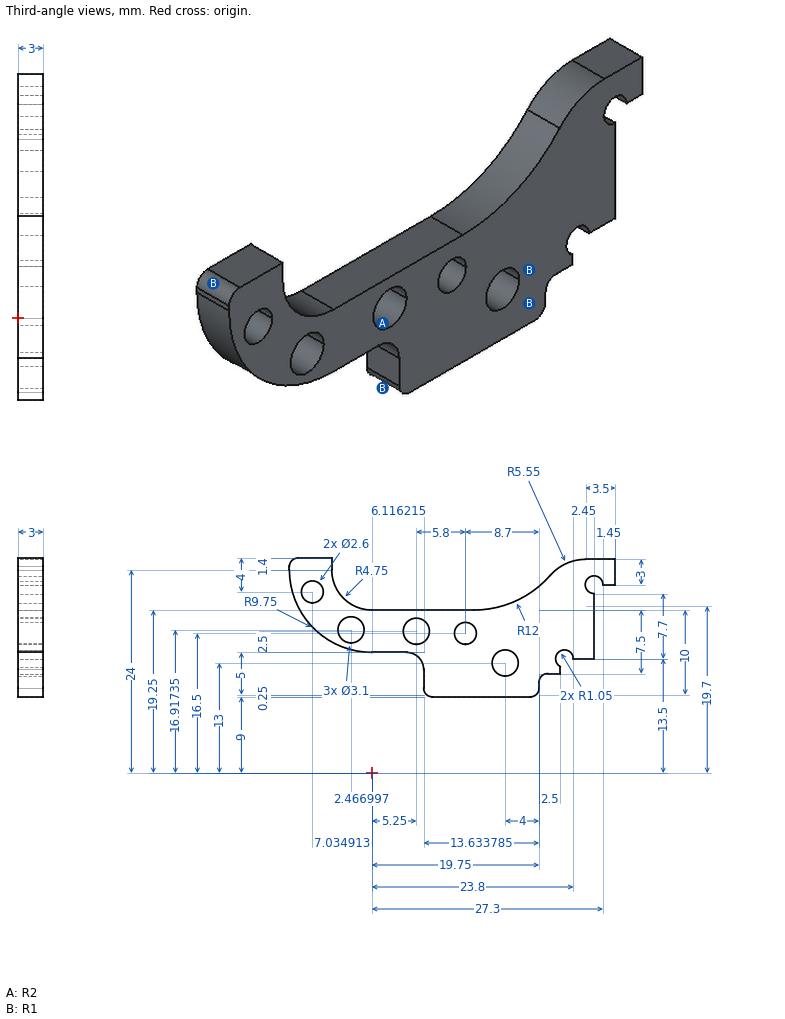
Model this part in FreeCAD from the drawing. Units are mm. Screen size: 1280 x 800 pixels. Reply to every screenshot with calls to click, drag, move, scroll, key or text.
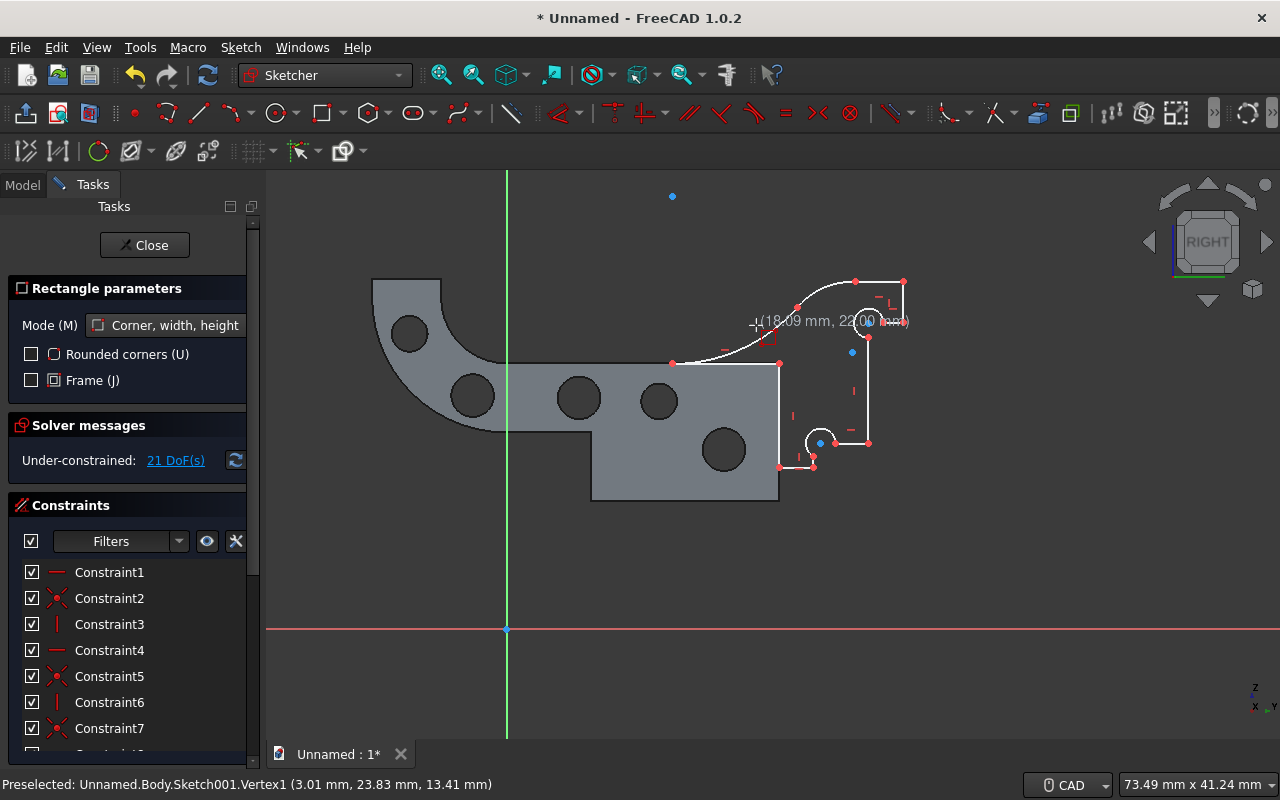
scroll(591, 501, up, 8)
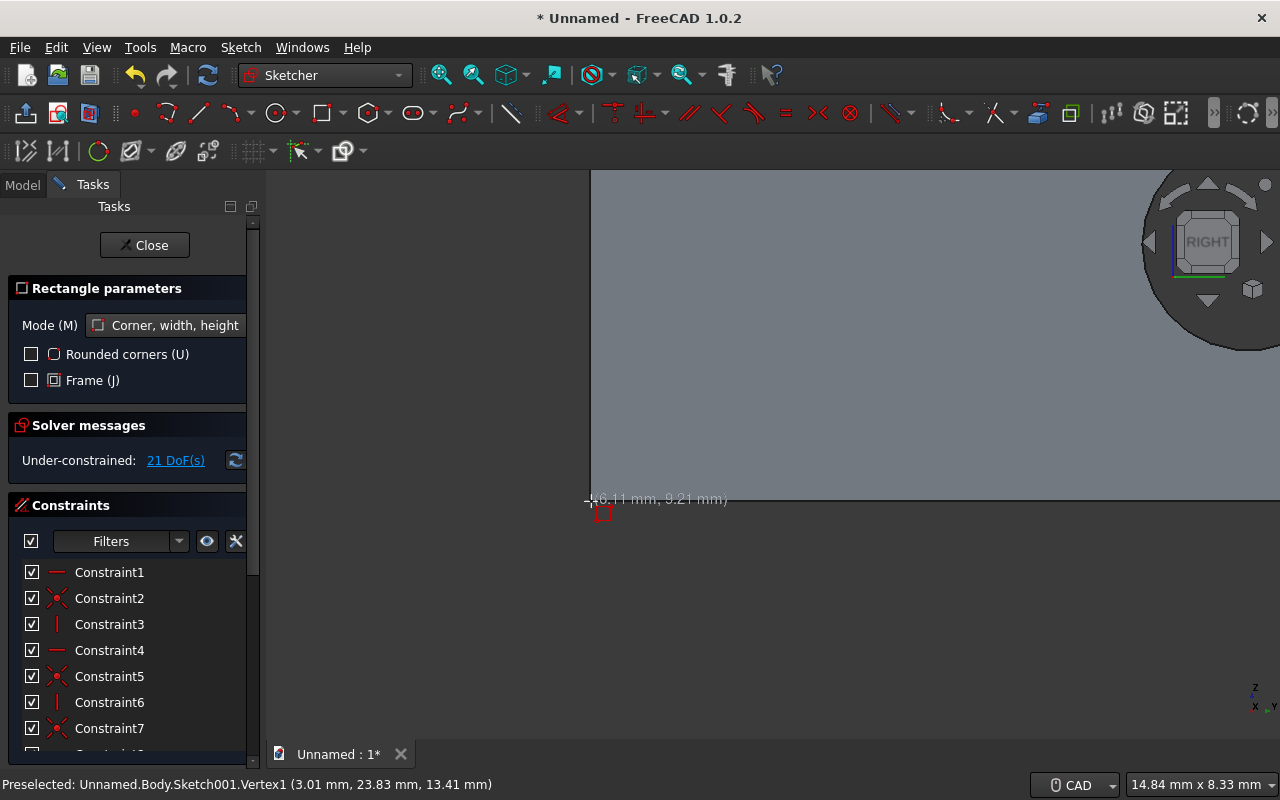
scroll(591, 501, down, 8)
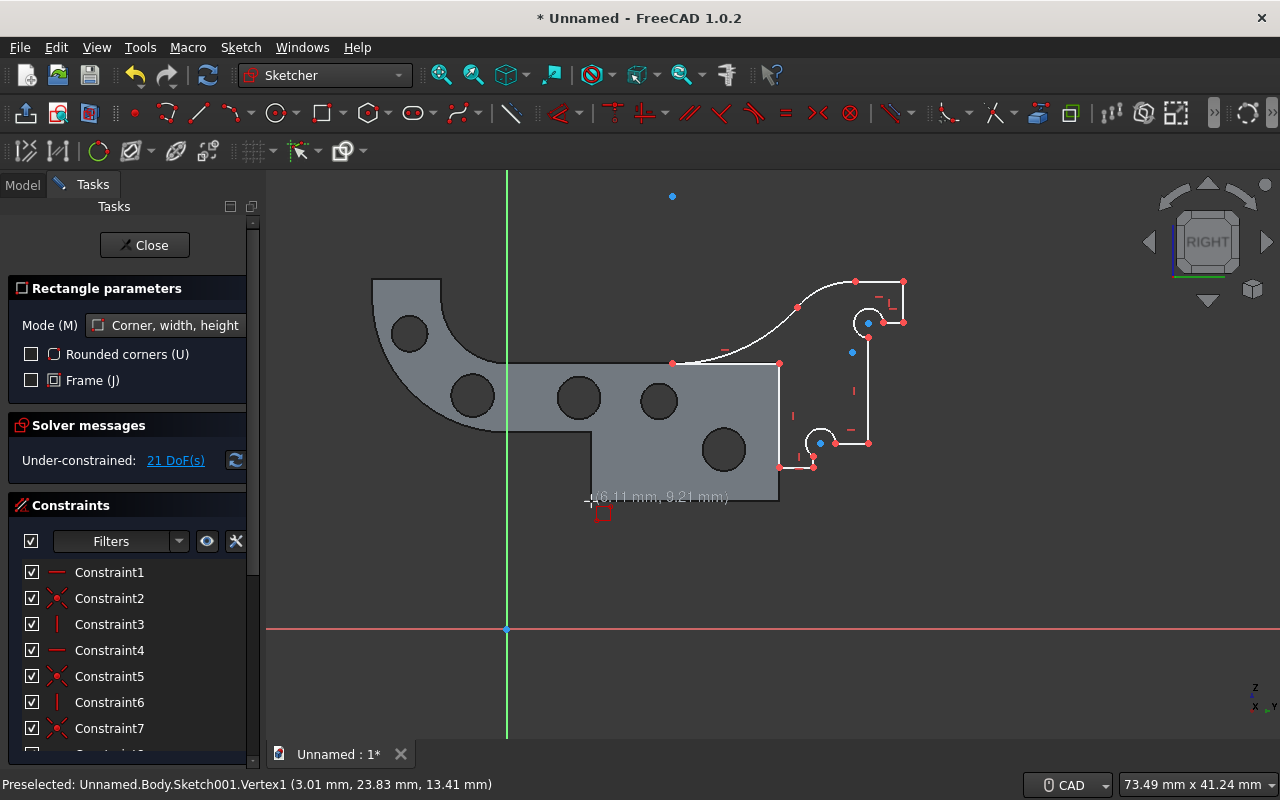
click(591, 501)
click(779, 505)
key(Escape)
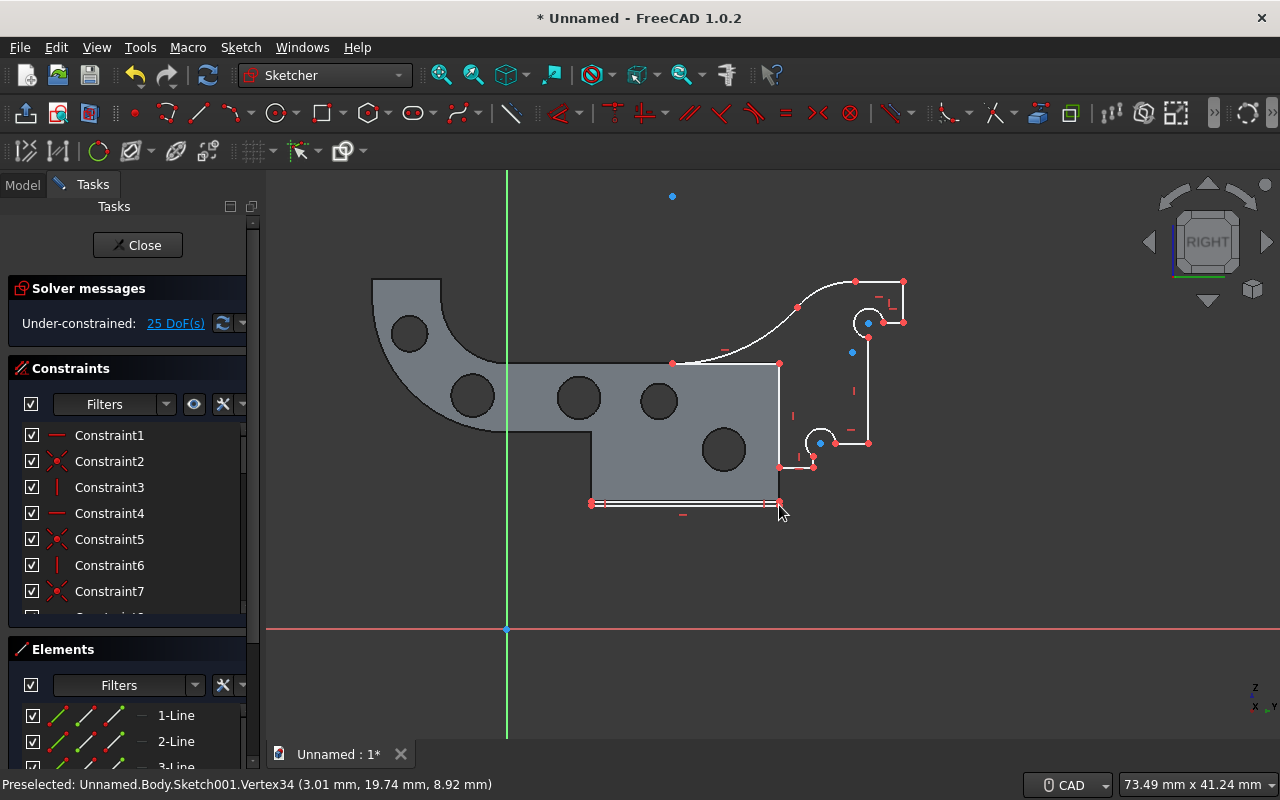
click(889, 282)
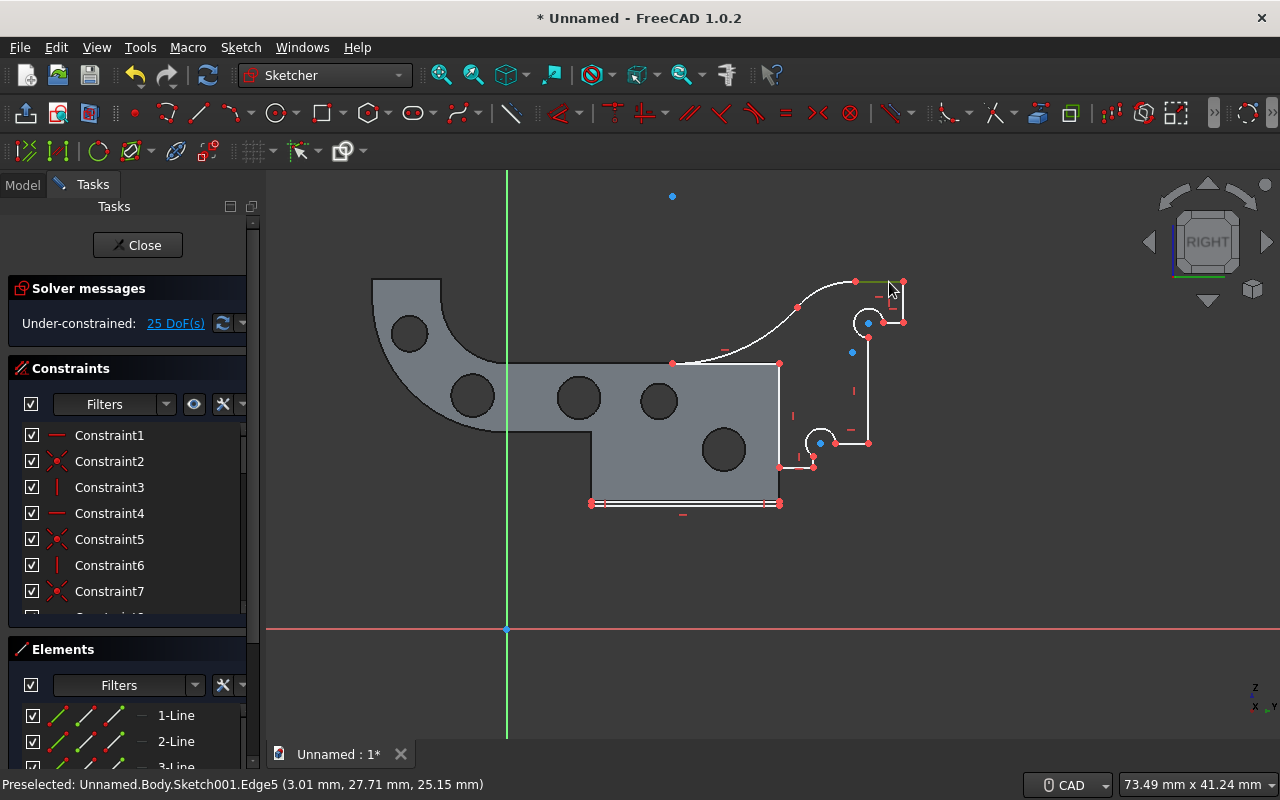
click(836, 284)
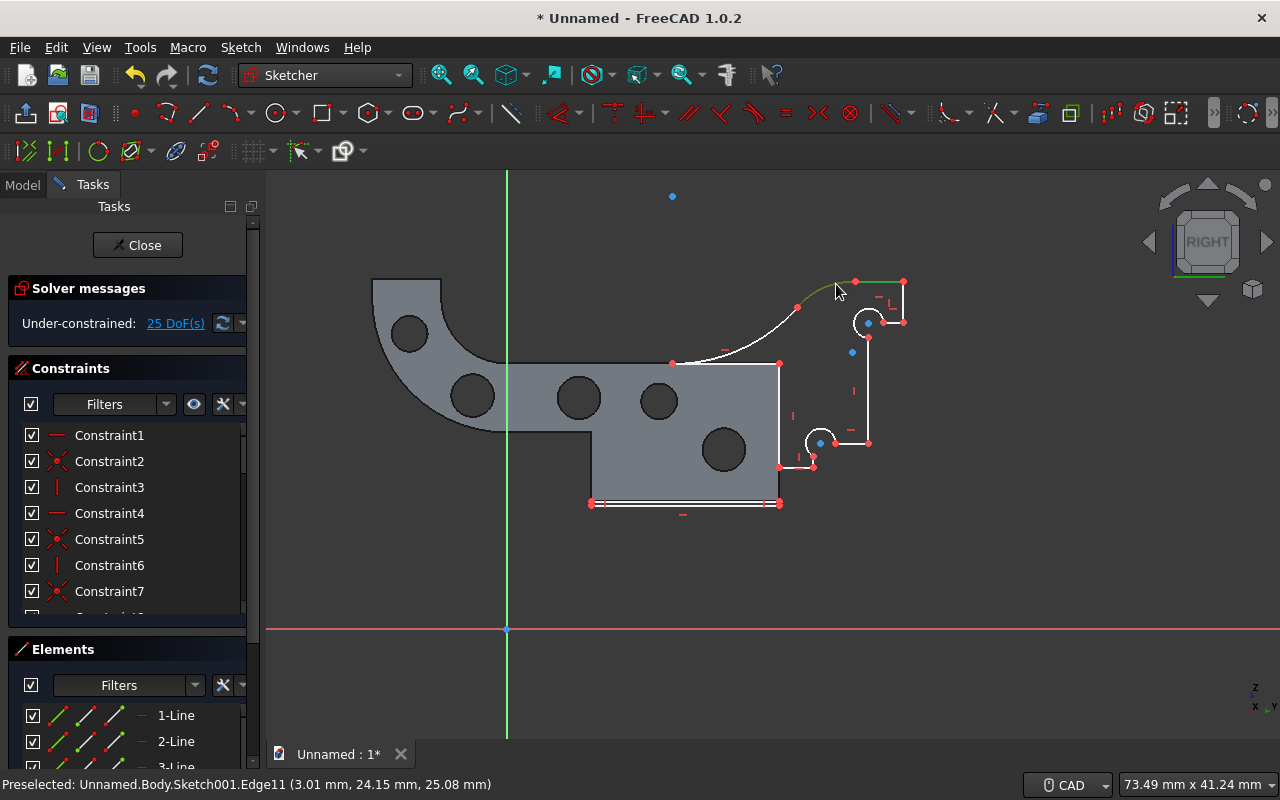
key(t)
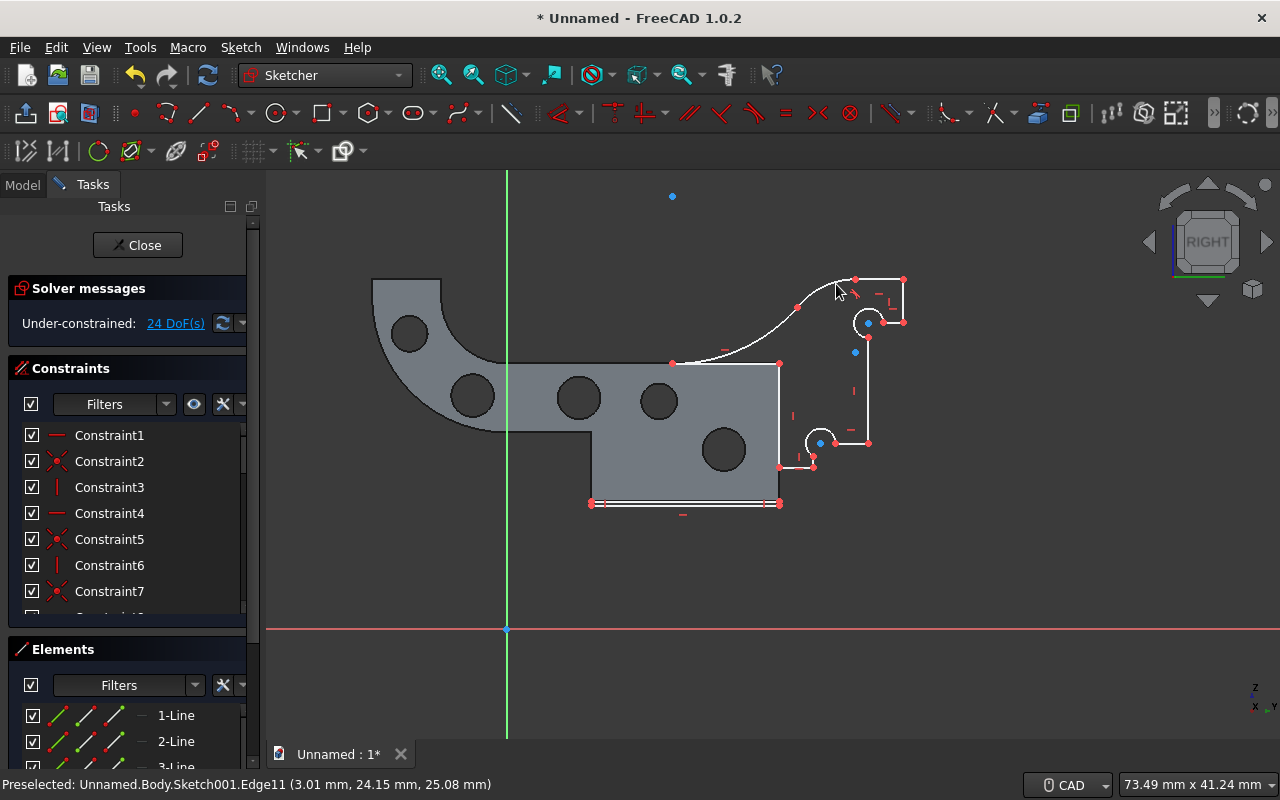
click(747, 364)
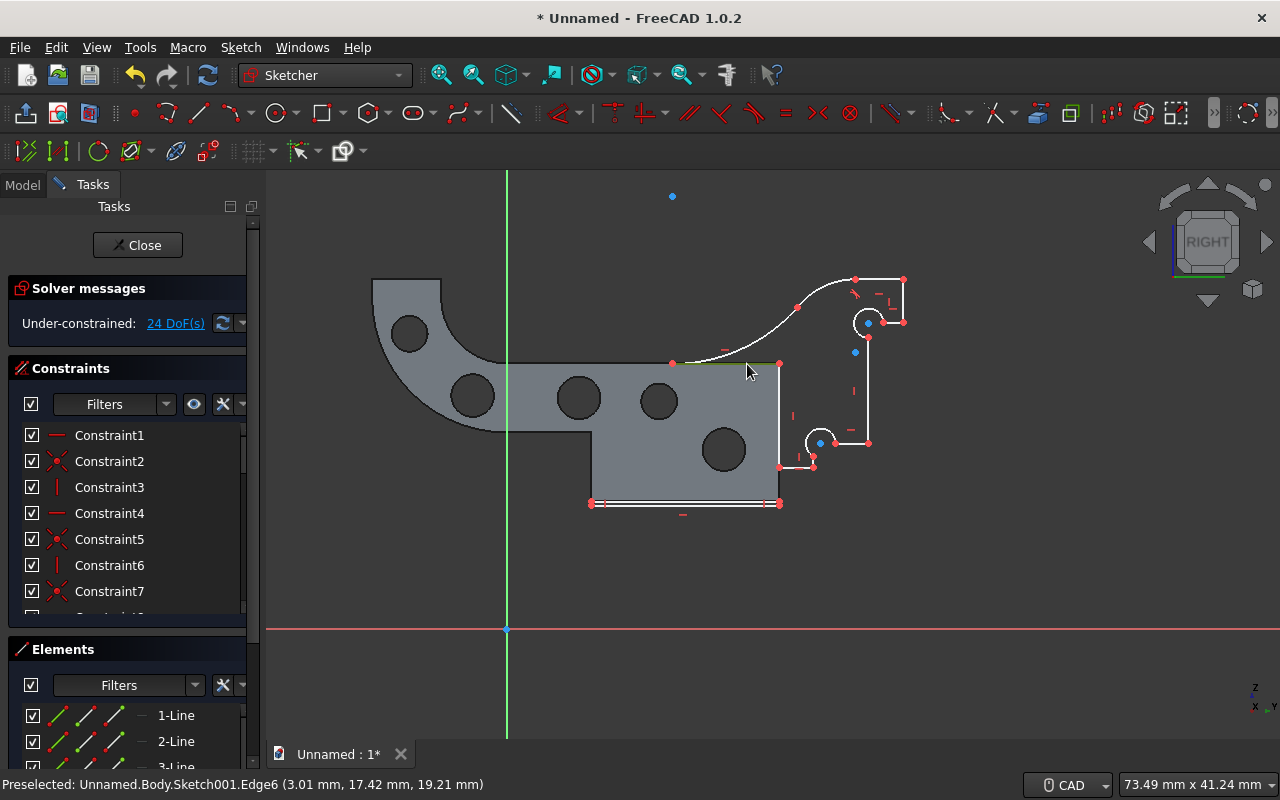
click(766, 335)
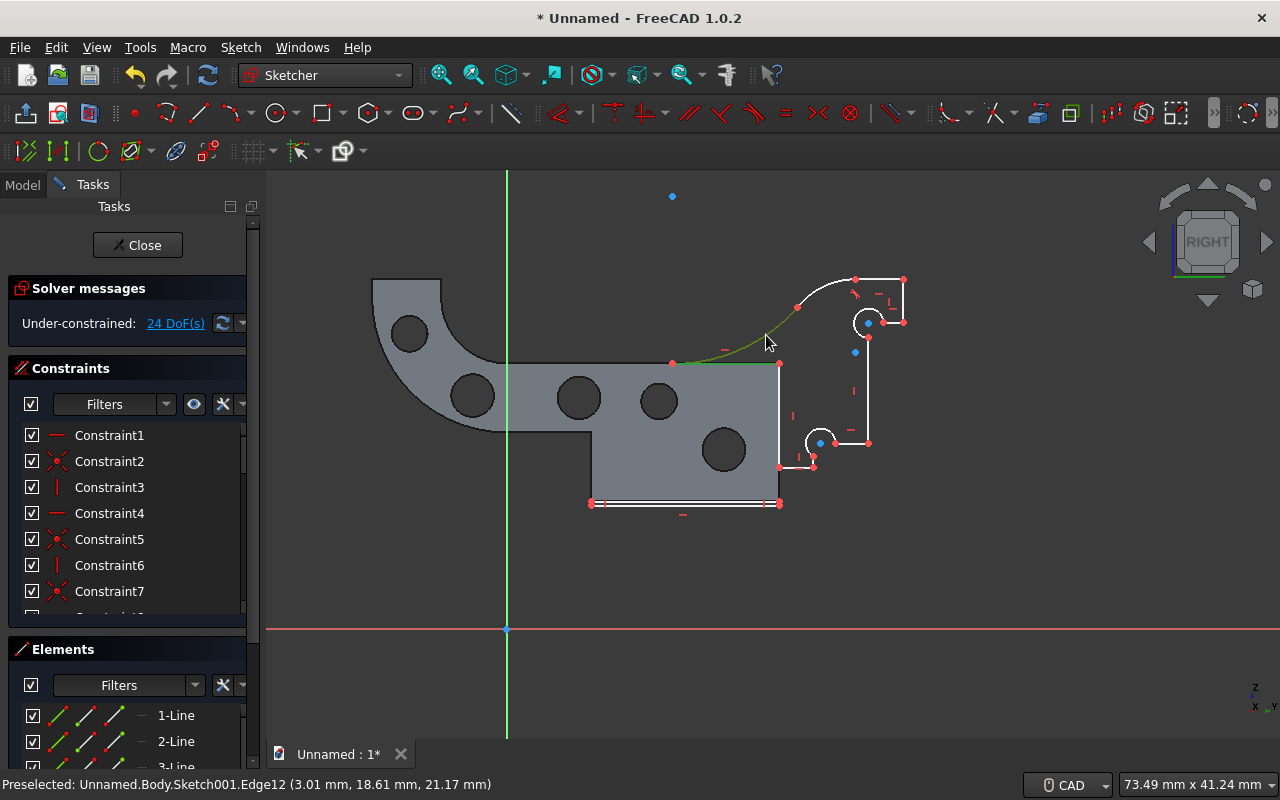
key(t)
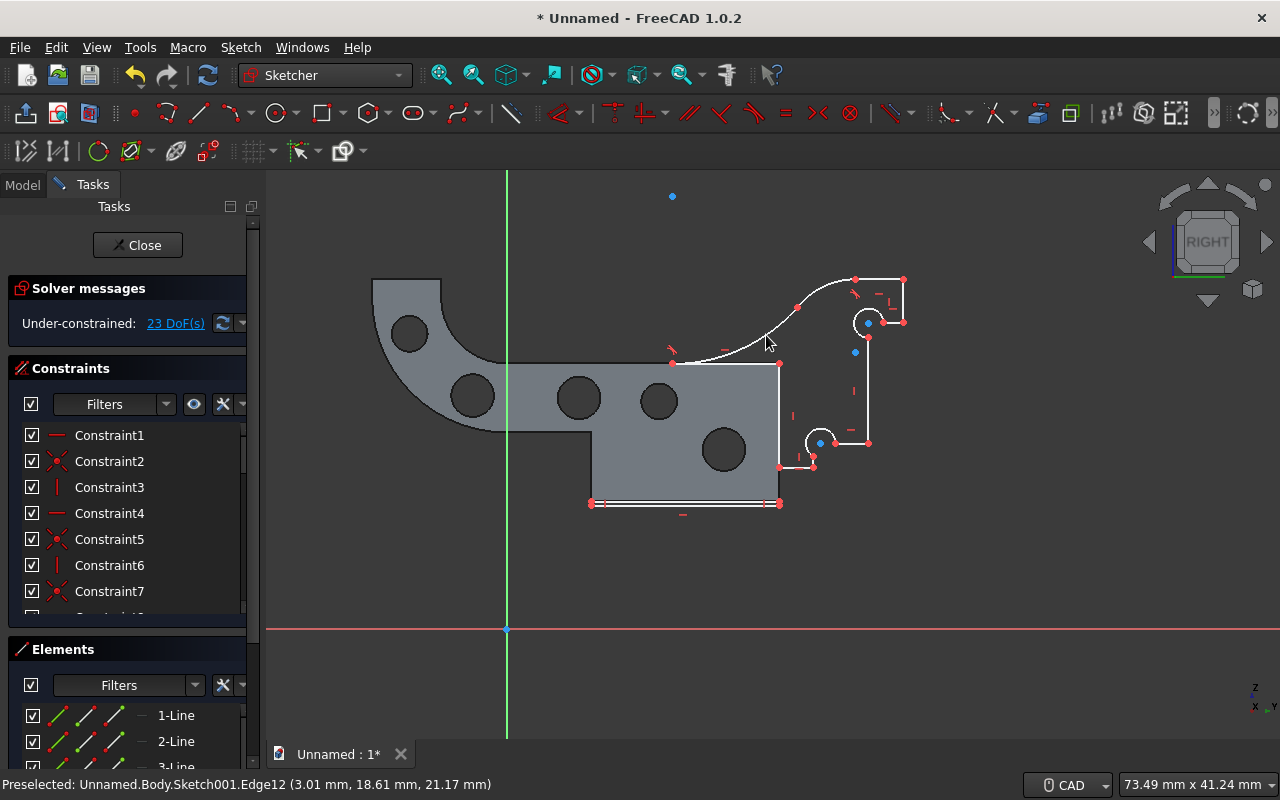
click(836, 282)